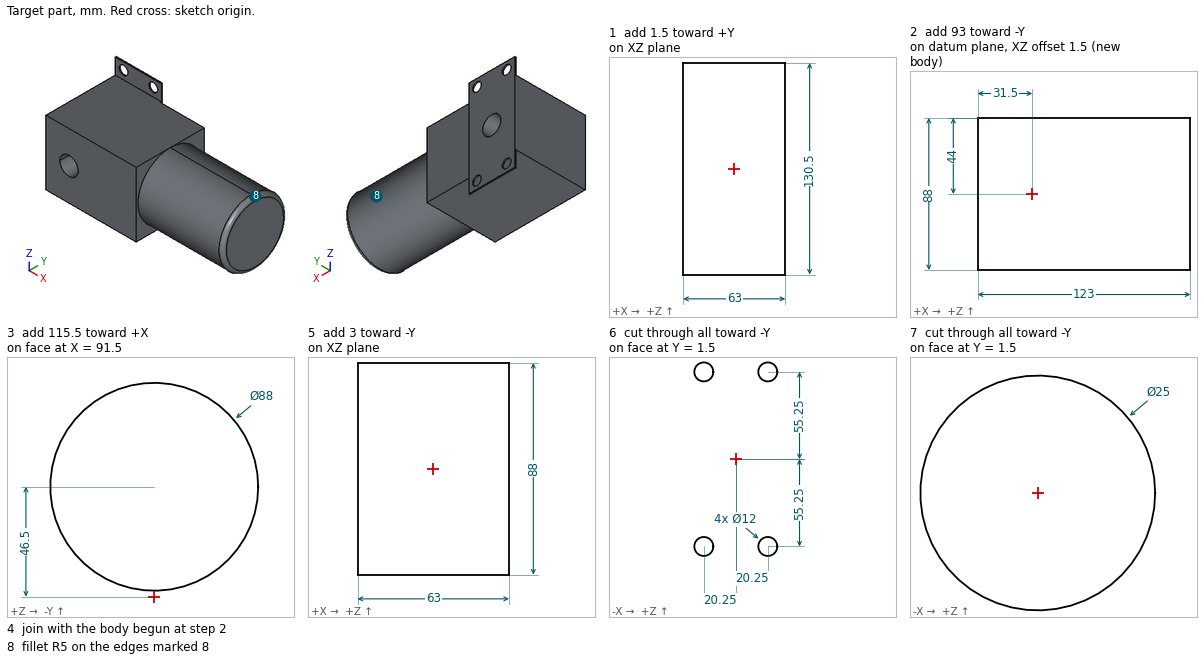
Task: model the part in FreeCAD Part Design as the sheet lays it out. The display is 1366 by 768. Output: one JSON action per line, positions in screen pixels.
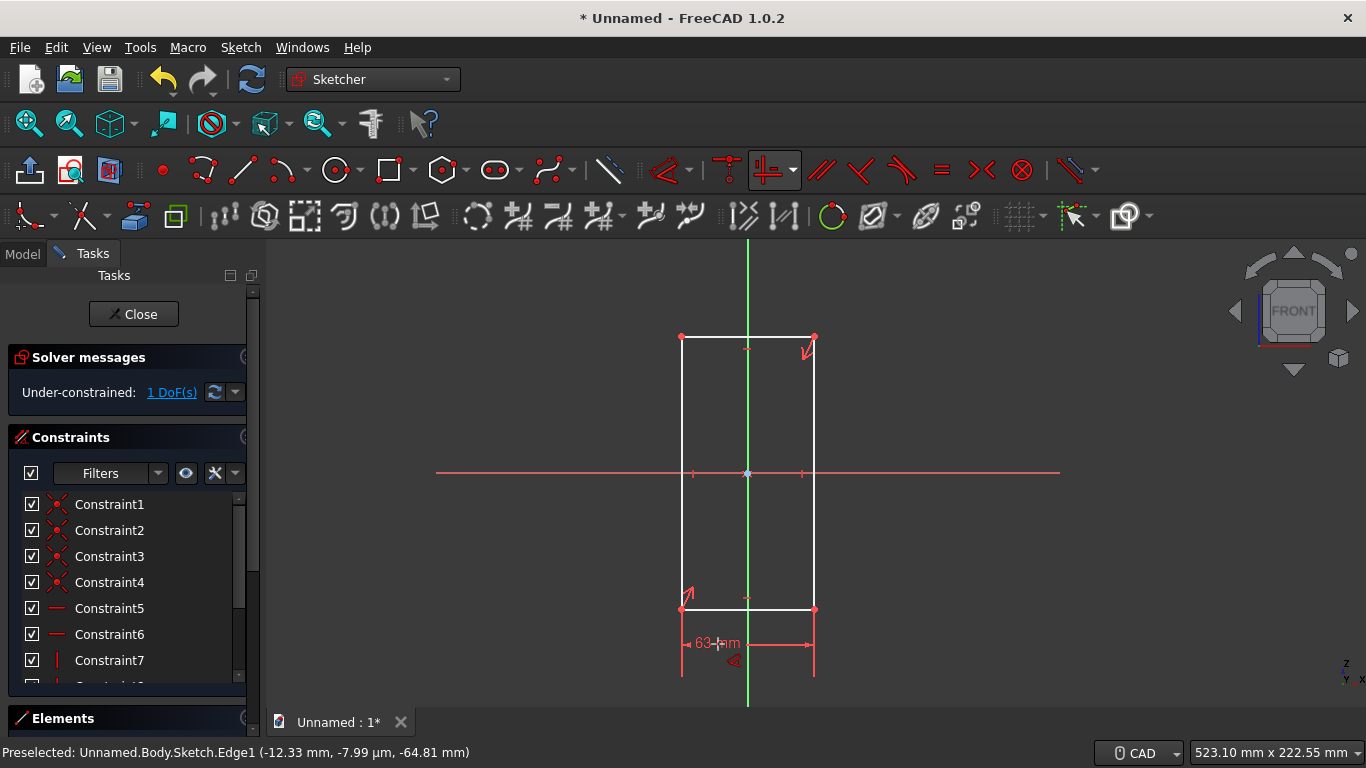
{"action": "left_click", "coordinate": [814, 528]}
{"action": "left_click", "coordinate": [848, 411]}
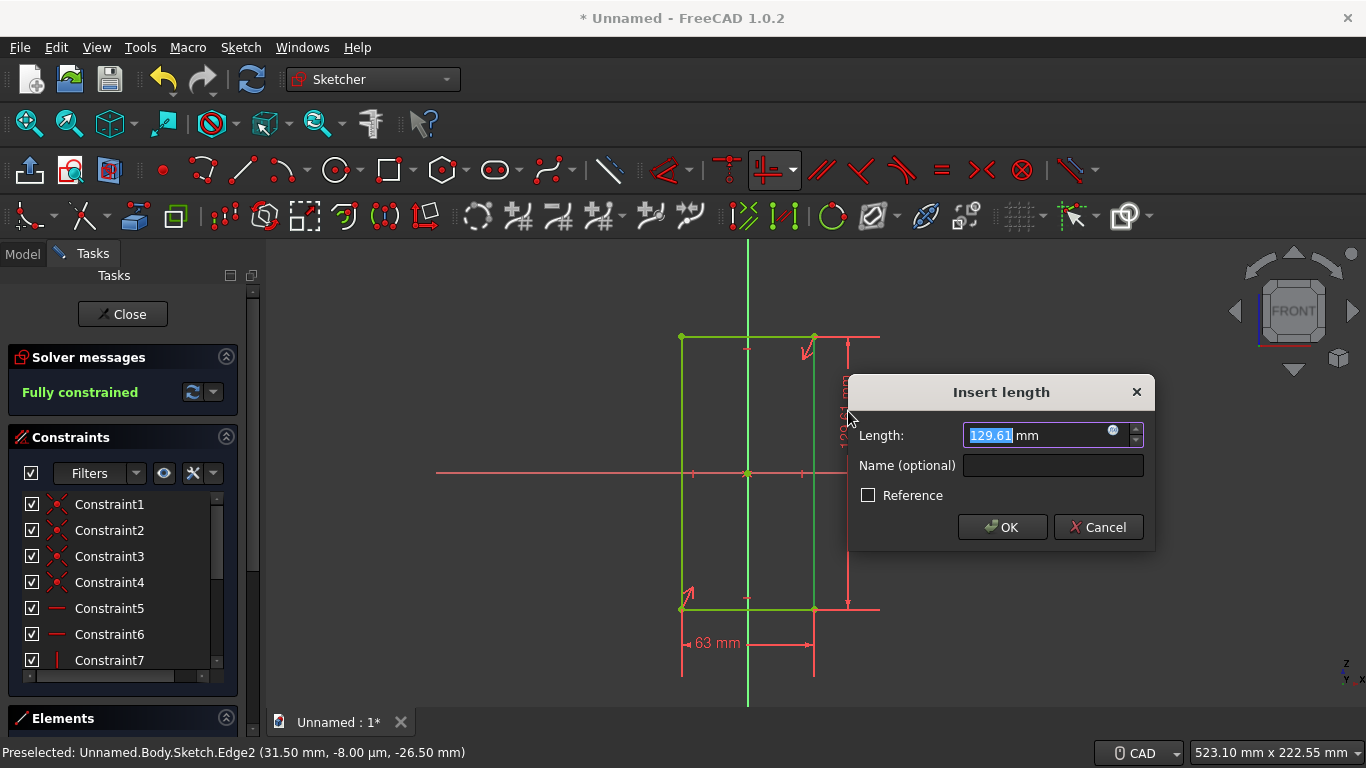
{"action": "type", "text": "130.5"}
{"action": "key", "text": "Return"}
{"action": "key", "text": "Escape"}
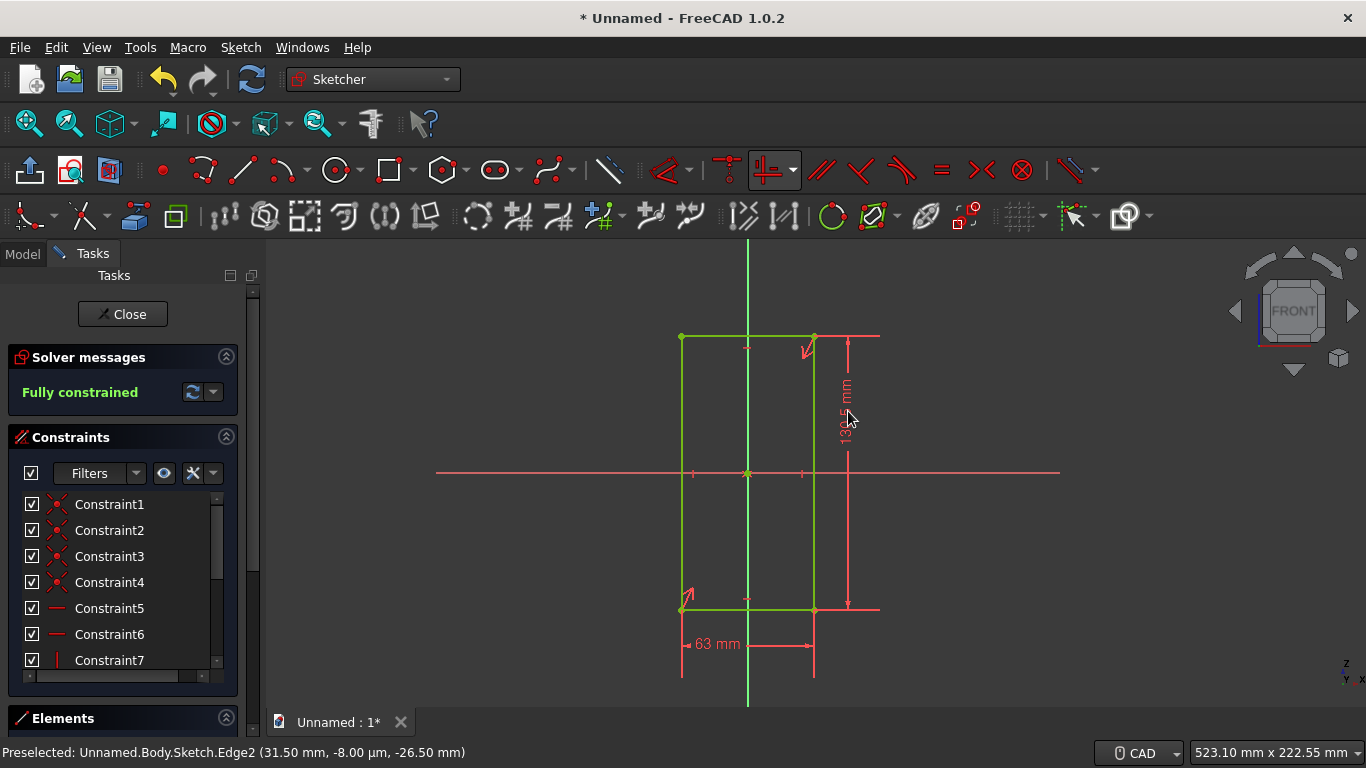
{"action": "left_click", "coordinate": [123, 314]}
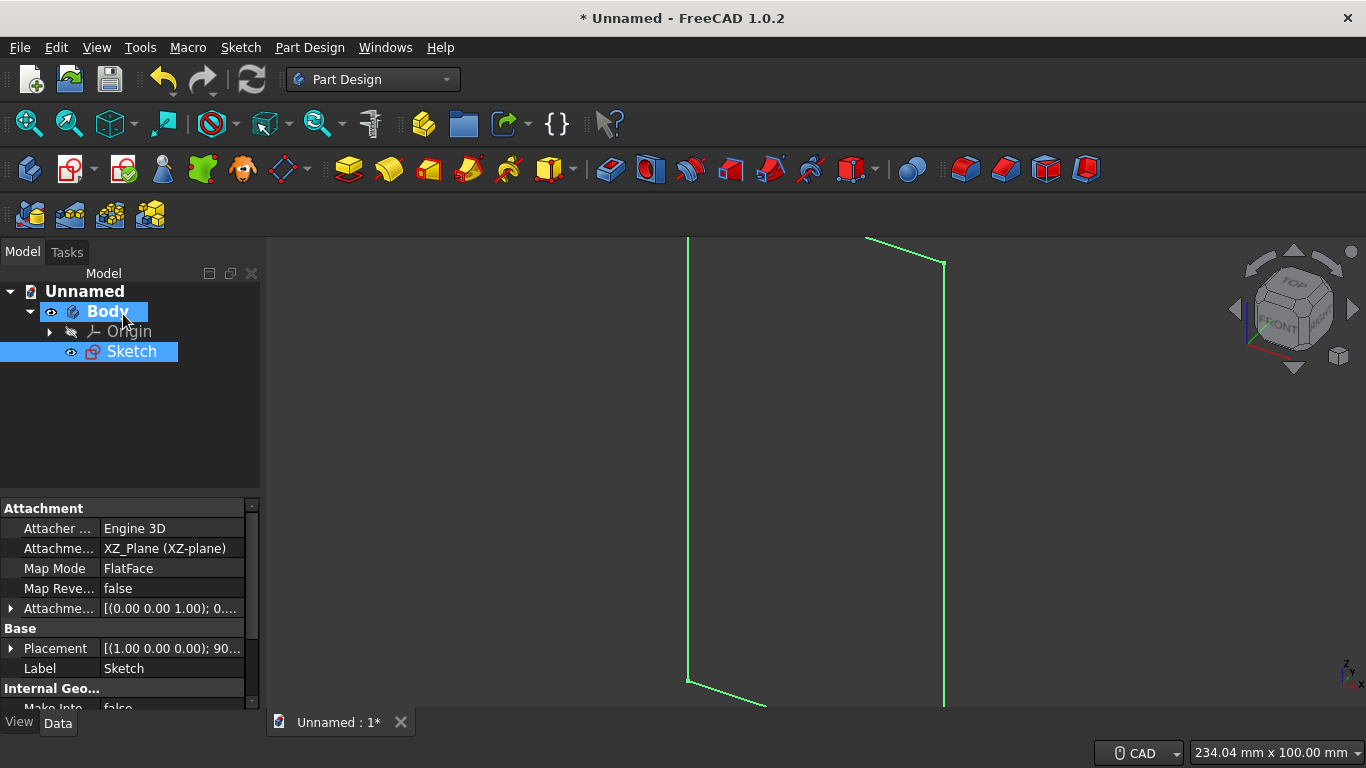
{"action": "left_click", "coordinate": [350, 170]}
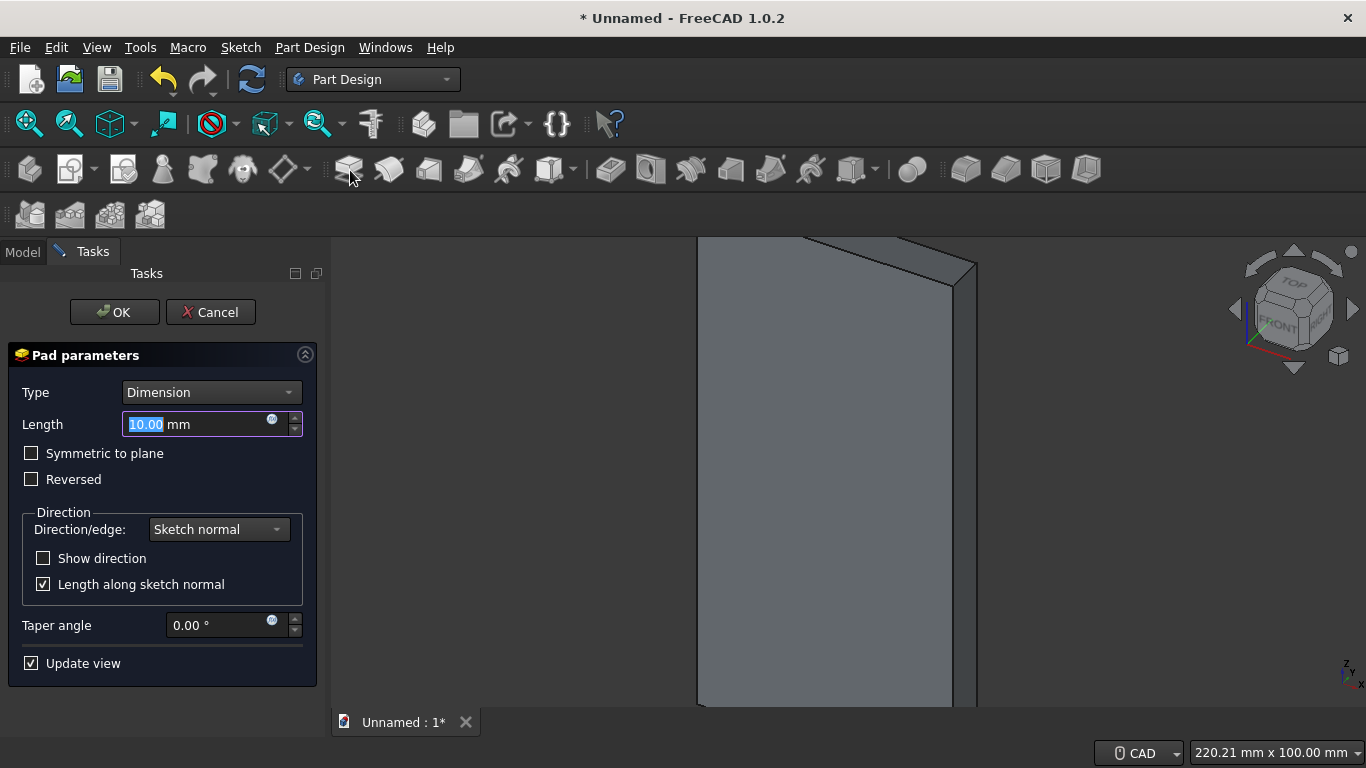
{"action": "type", "text": "1.5"}
{"action": "key", "text": "Tab"}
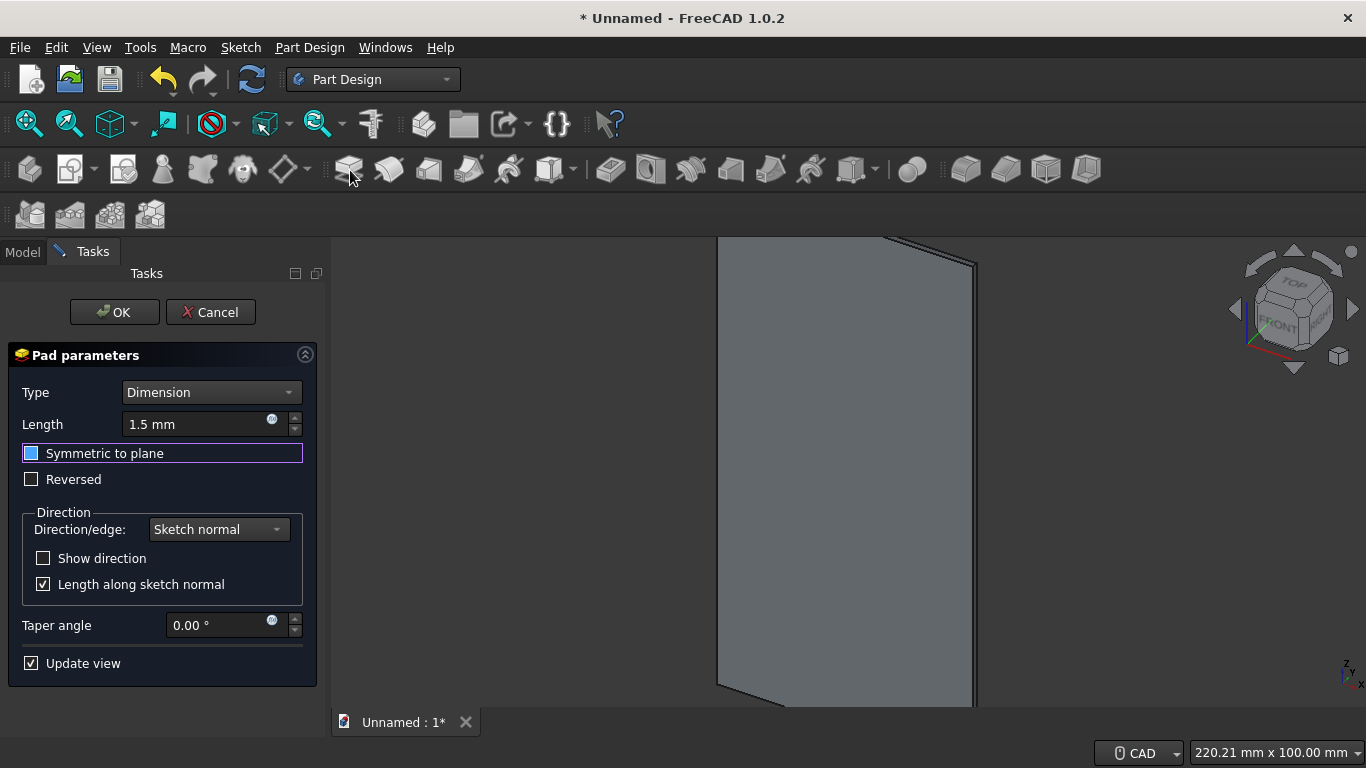
{"action": "left_click", "coordinate": [30, 479]}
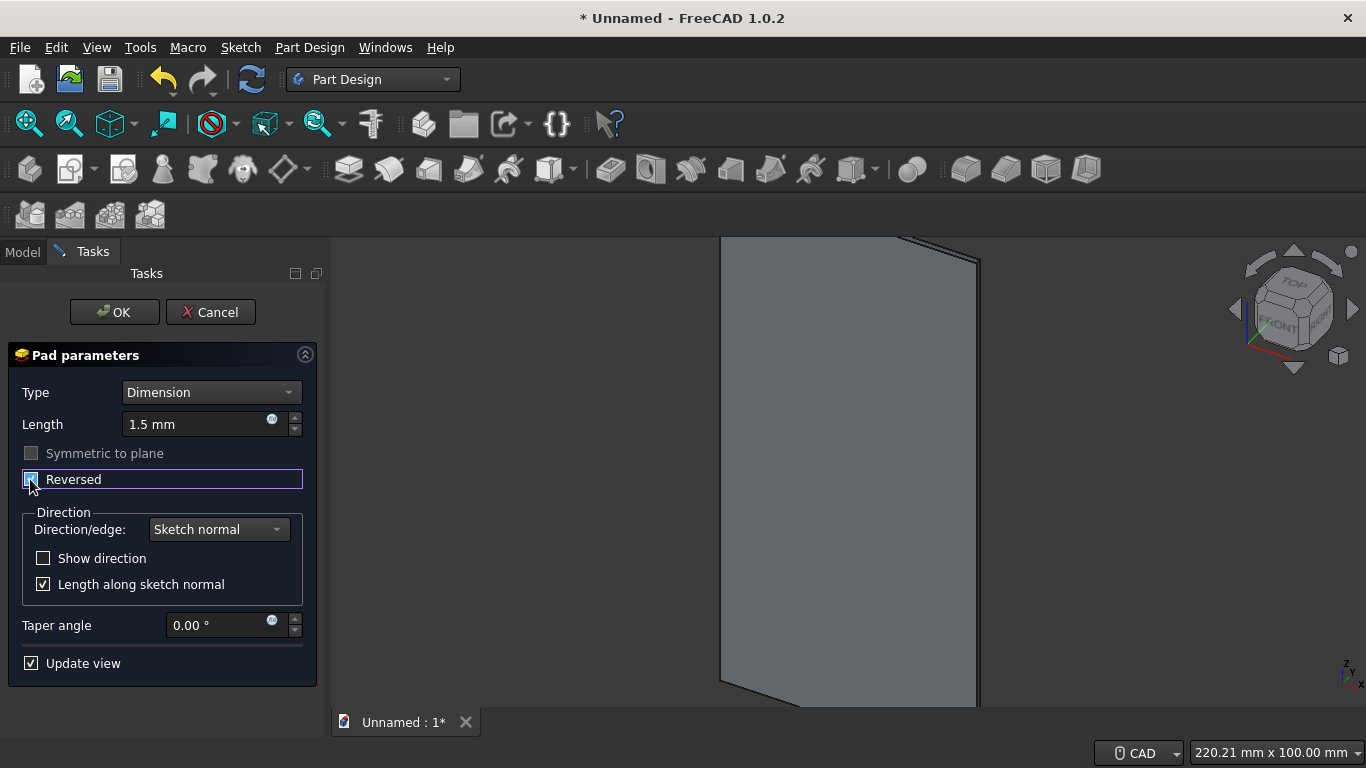
{"action": "left_click", "coordinate": [115, 312]}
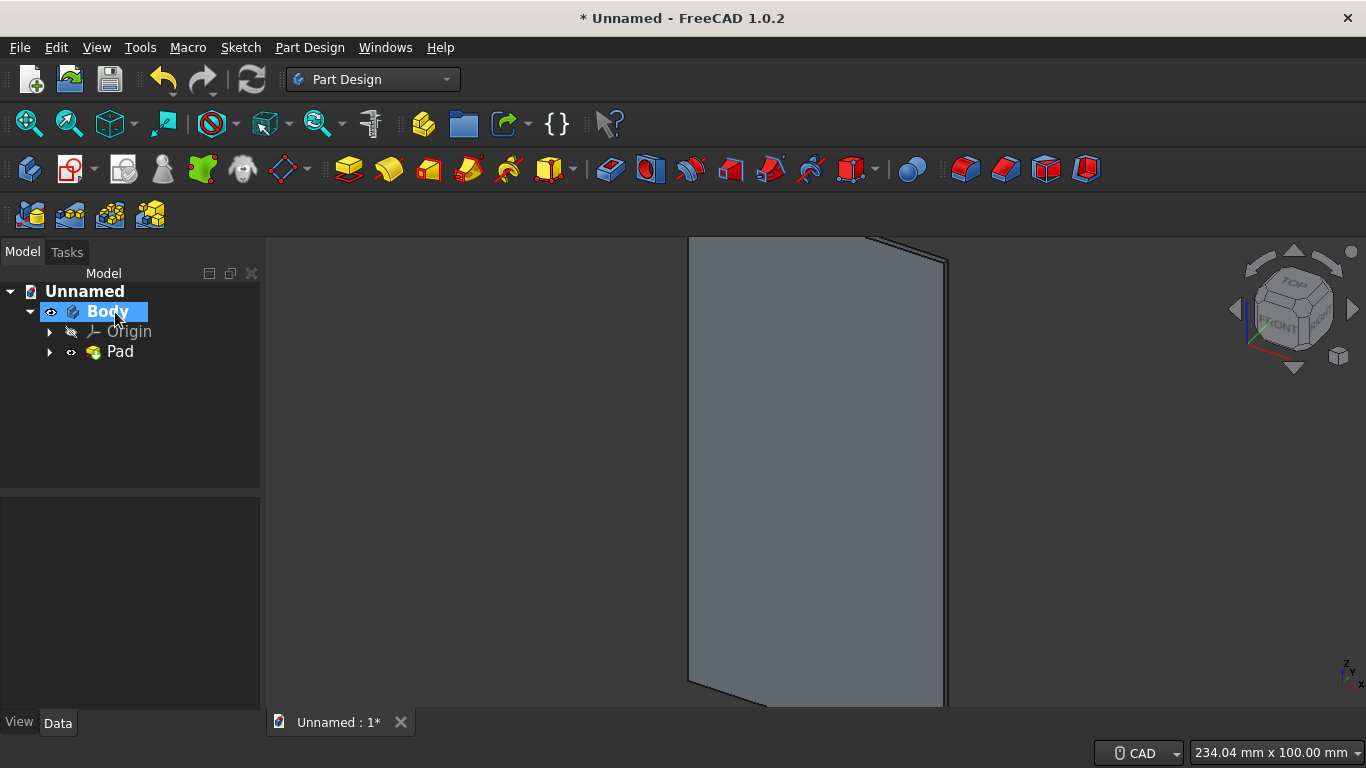
{"action": "left_click", "coordinate": [30, 124]}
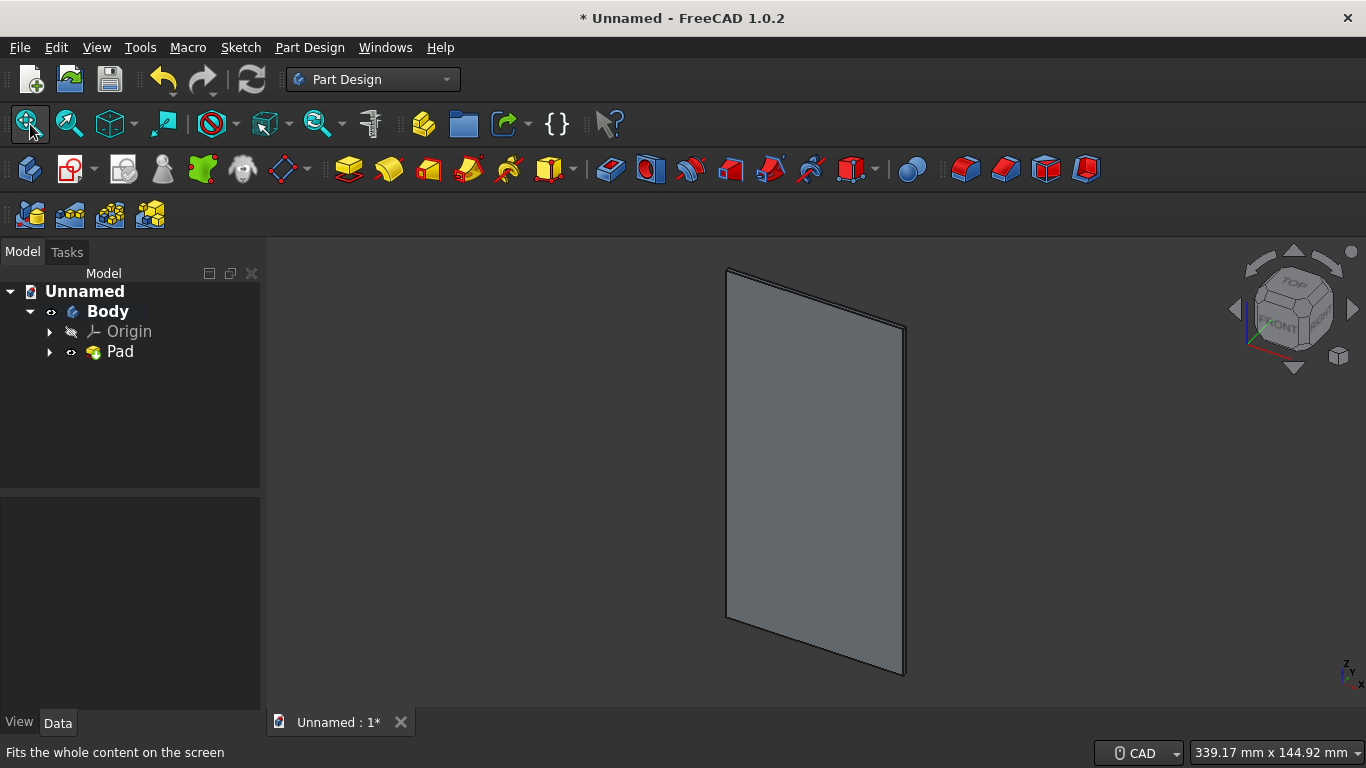
{"action": "left_click", "coordinate": [30, 170]}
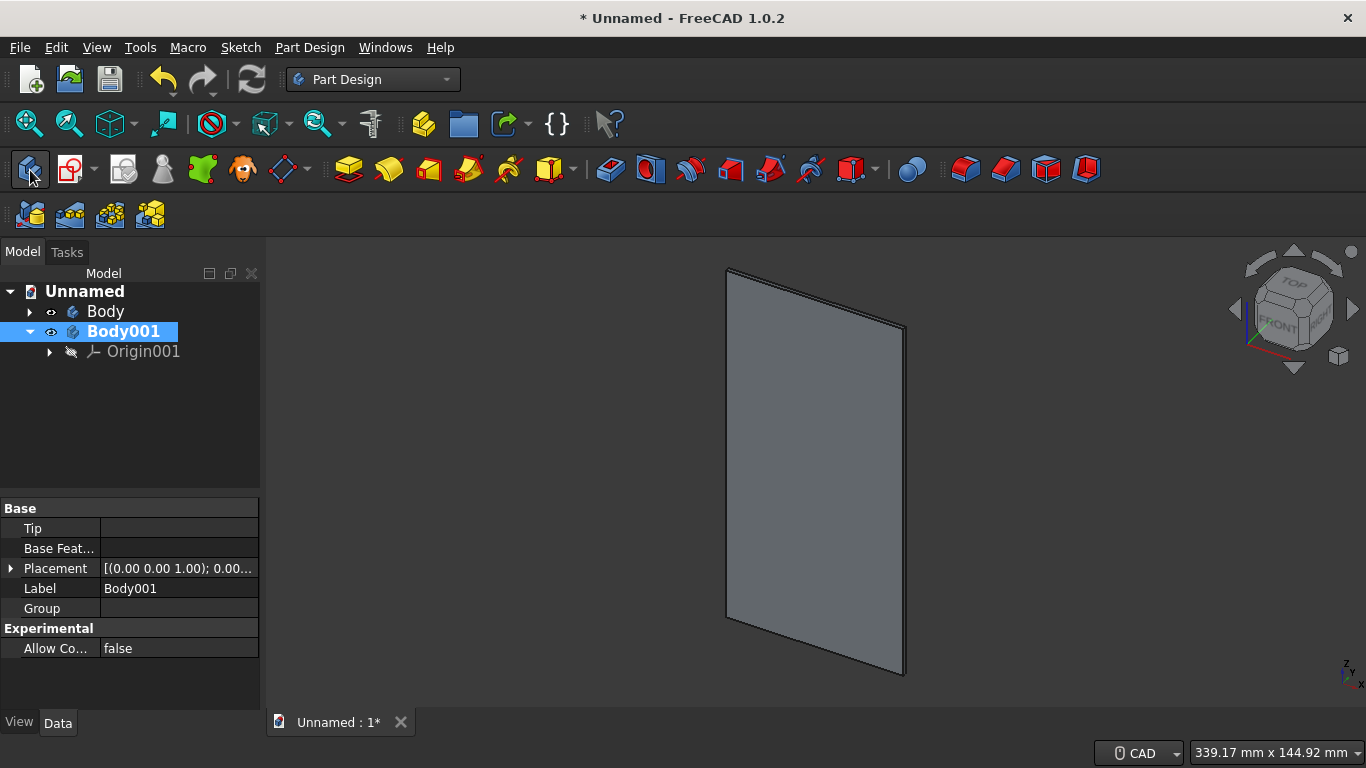
{"action": "left_click", "coordinate": [50, 352]}